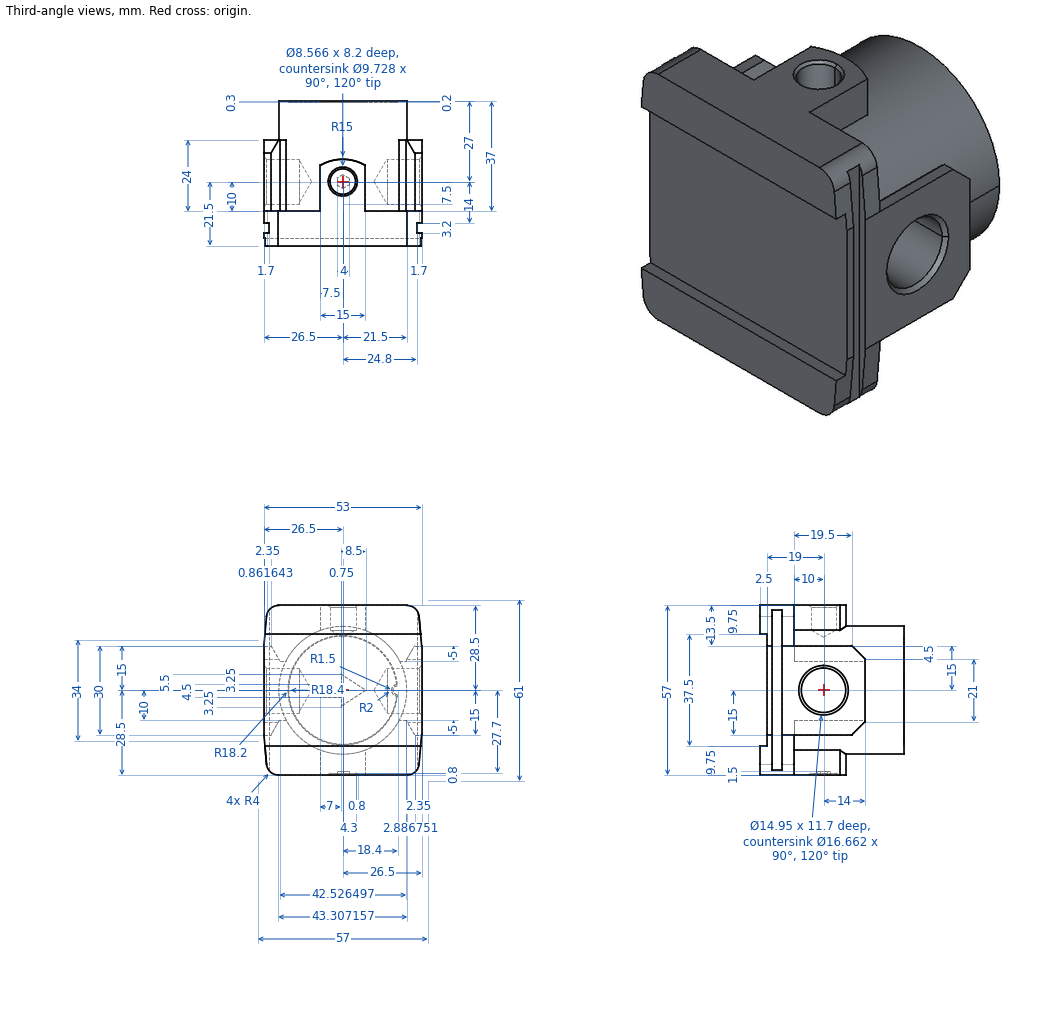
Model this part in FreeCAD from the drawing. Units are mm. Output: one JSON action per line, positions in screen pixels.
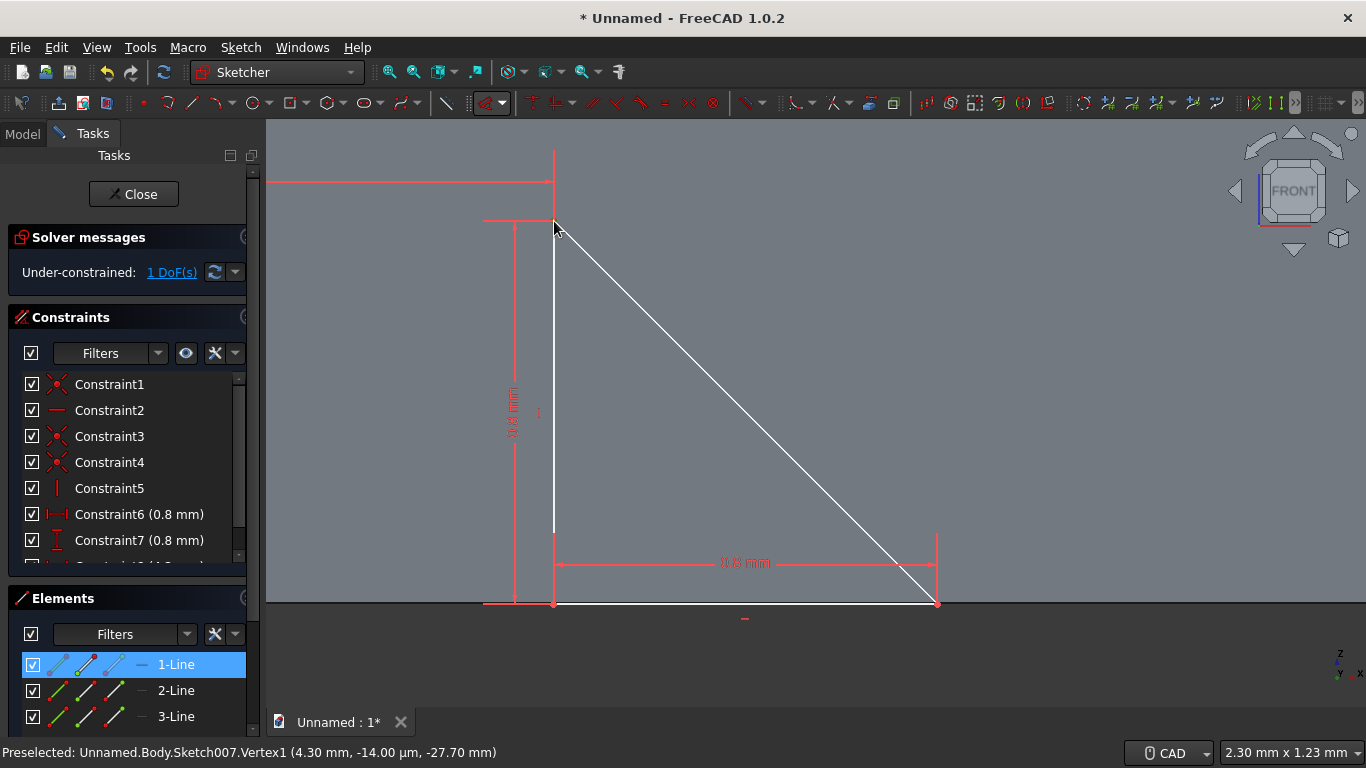
{"action": "left_click", "coordinate": [504, 104]}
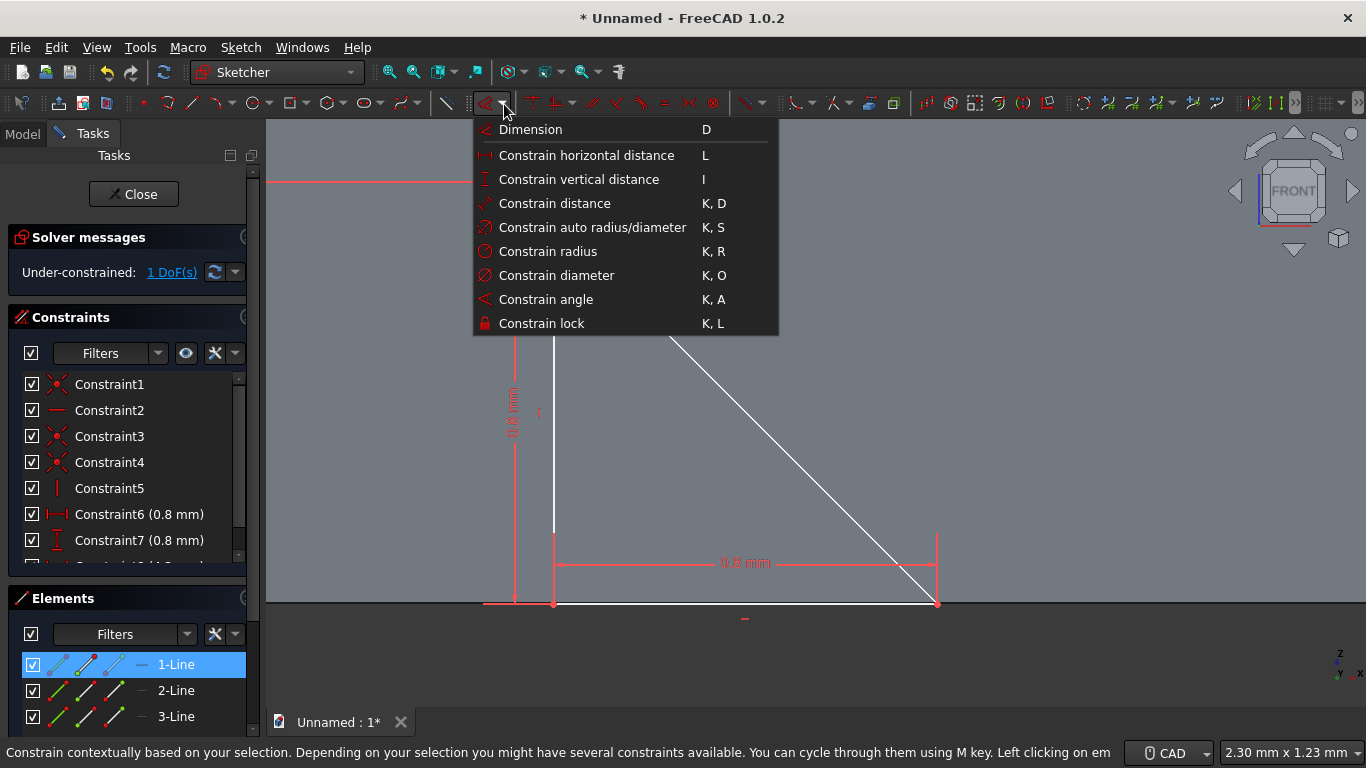
{"action": "left_click", "coordinate": [626, 179]}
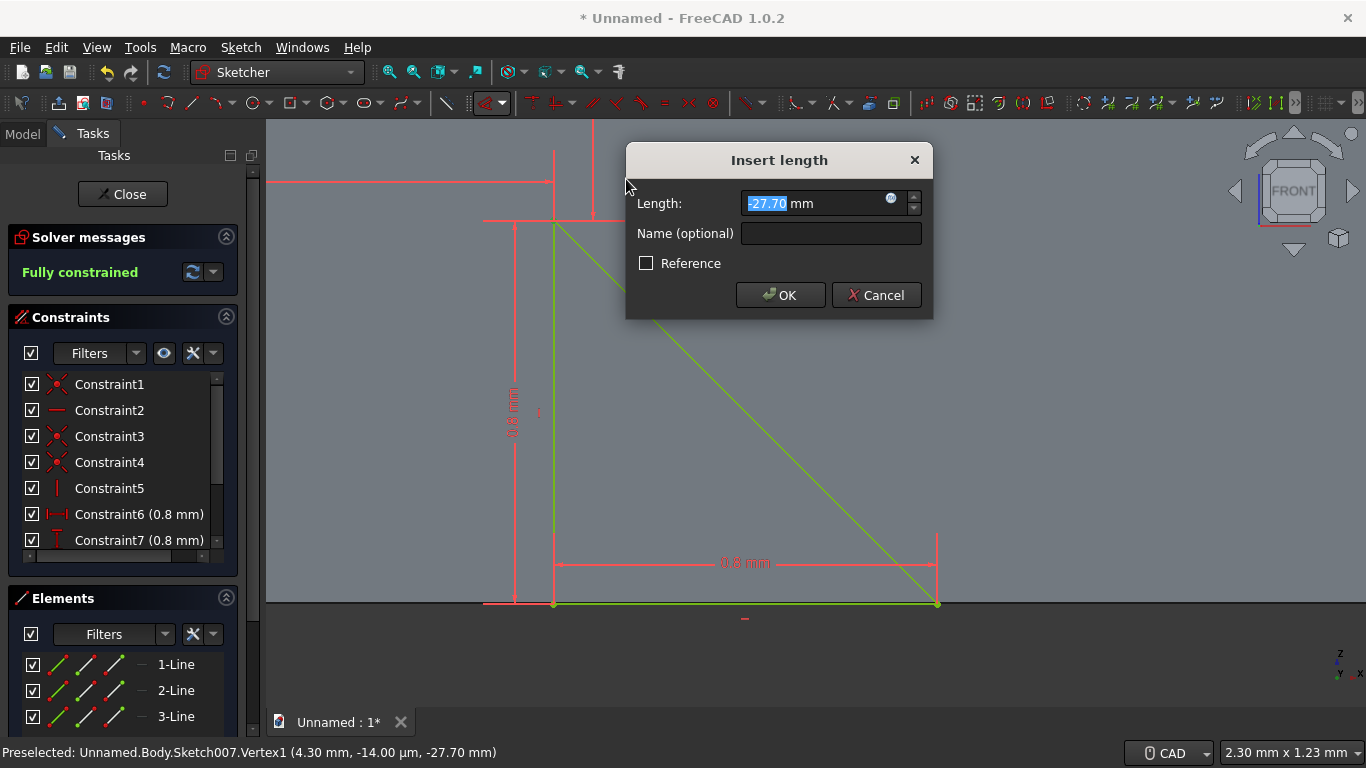
{"action": "type", "text": "-27.7"}
{"action": "key", "text": "Return"}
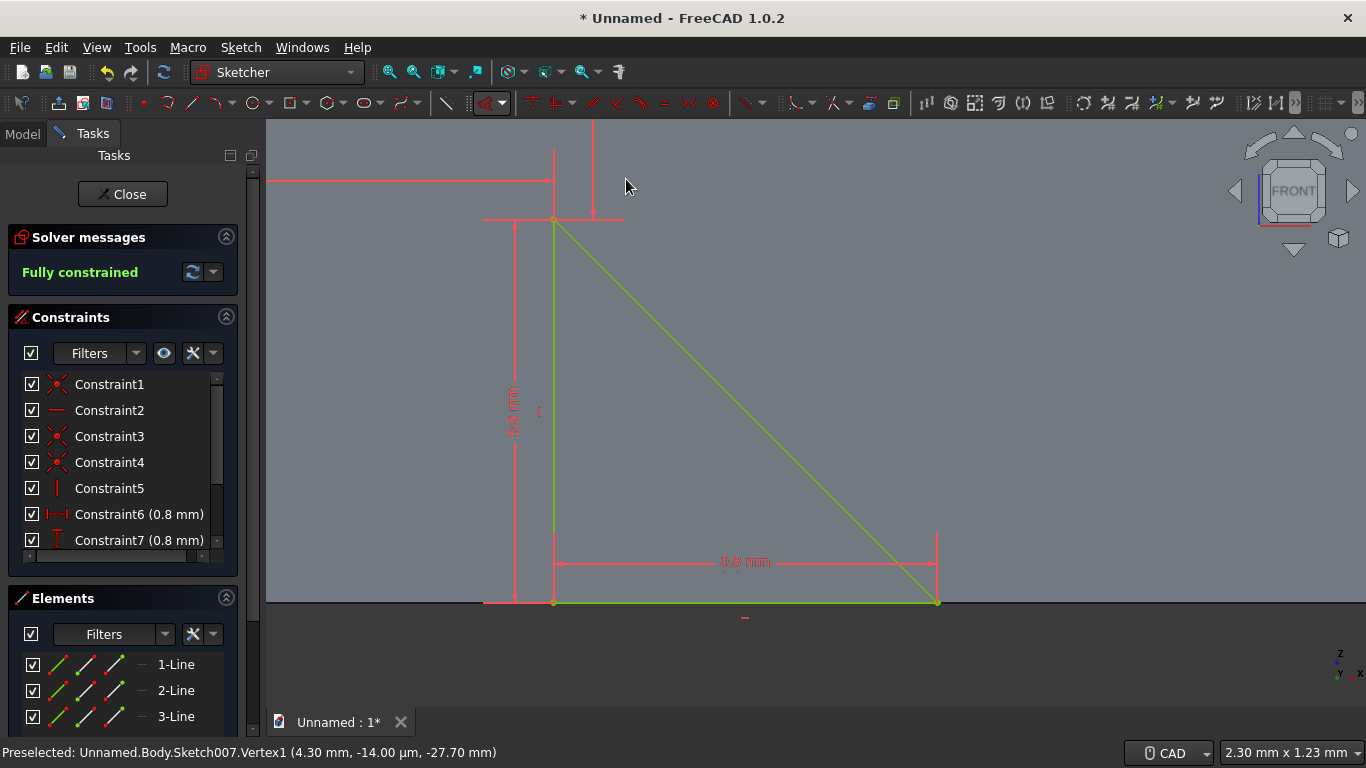
{"action": "left_click", "coordinate": [123, 194]}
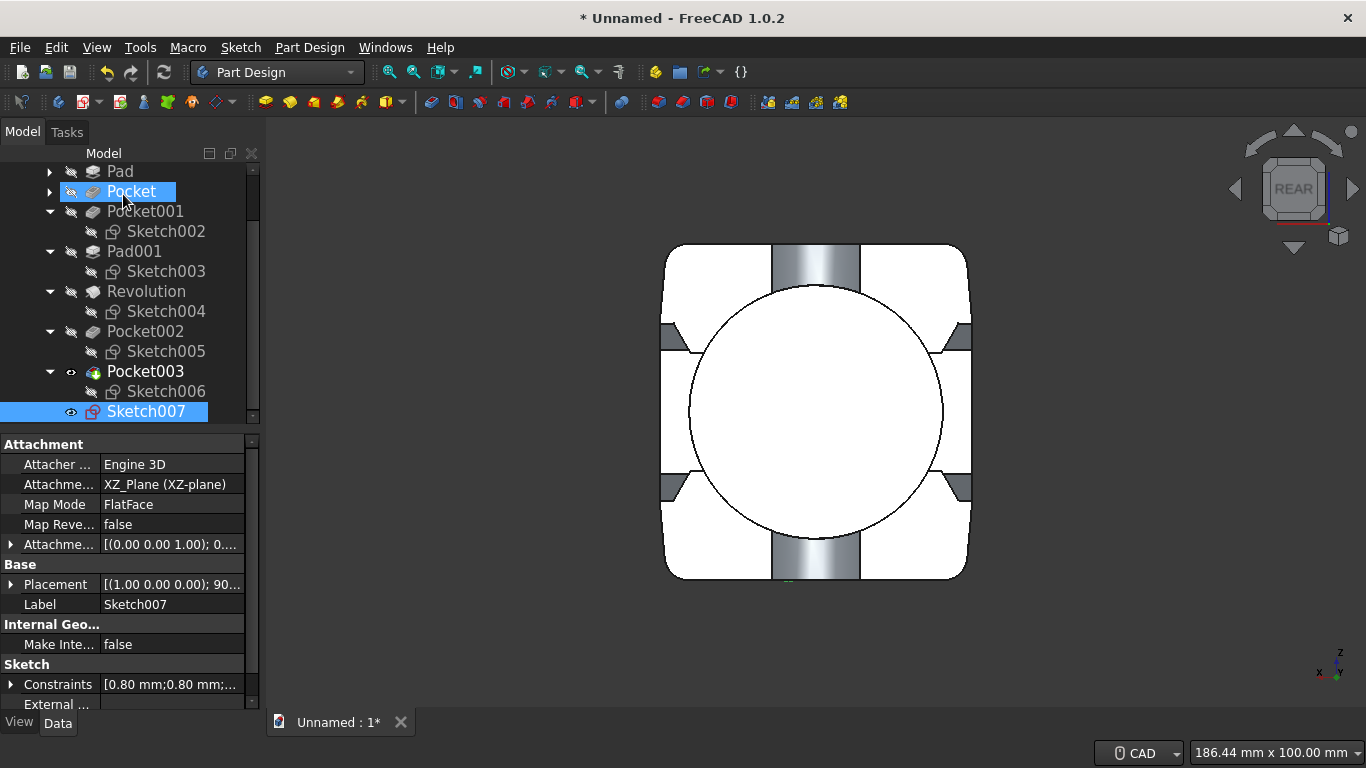
{"action": "left_click", "coordinate": [480, 102]}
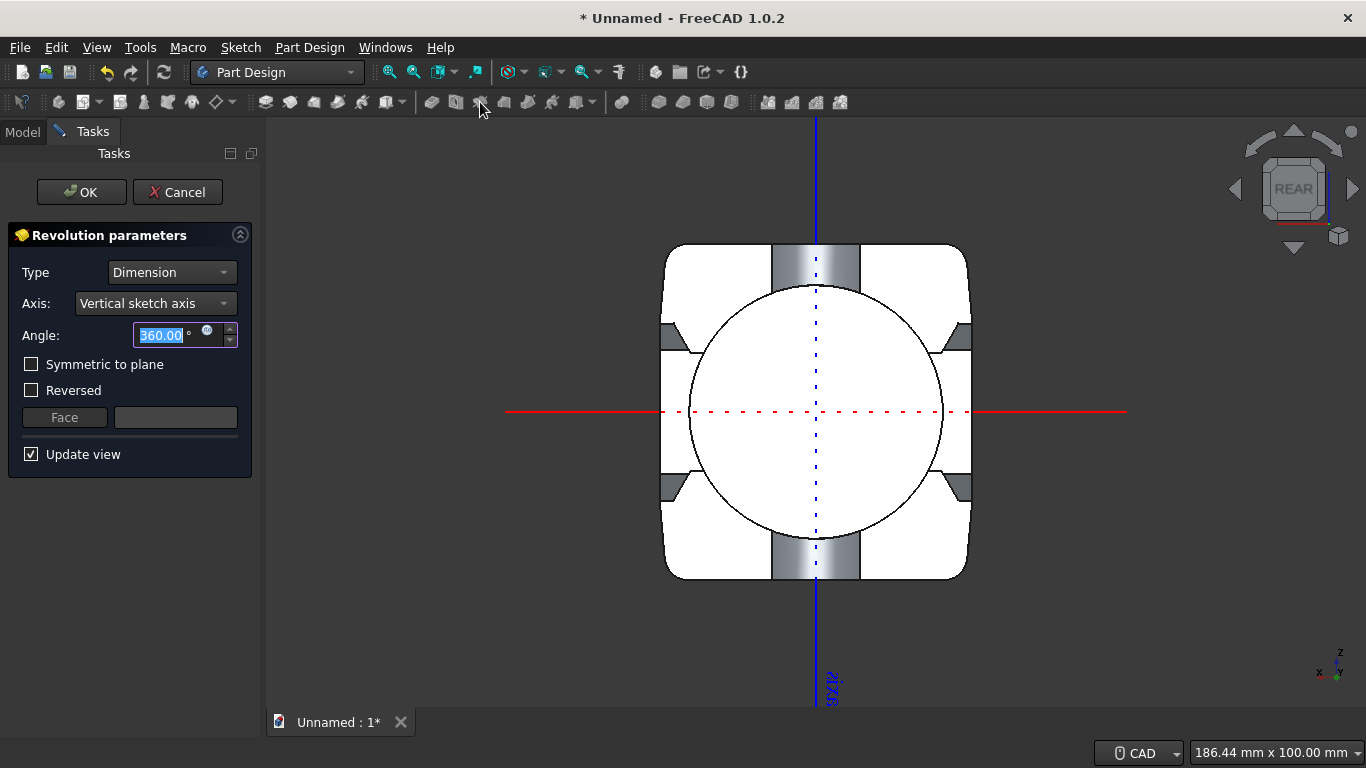
{"action": "left_click", "coordinate": [82, 192]}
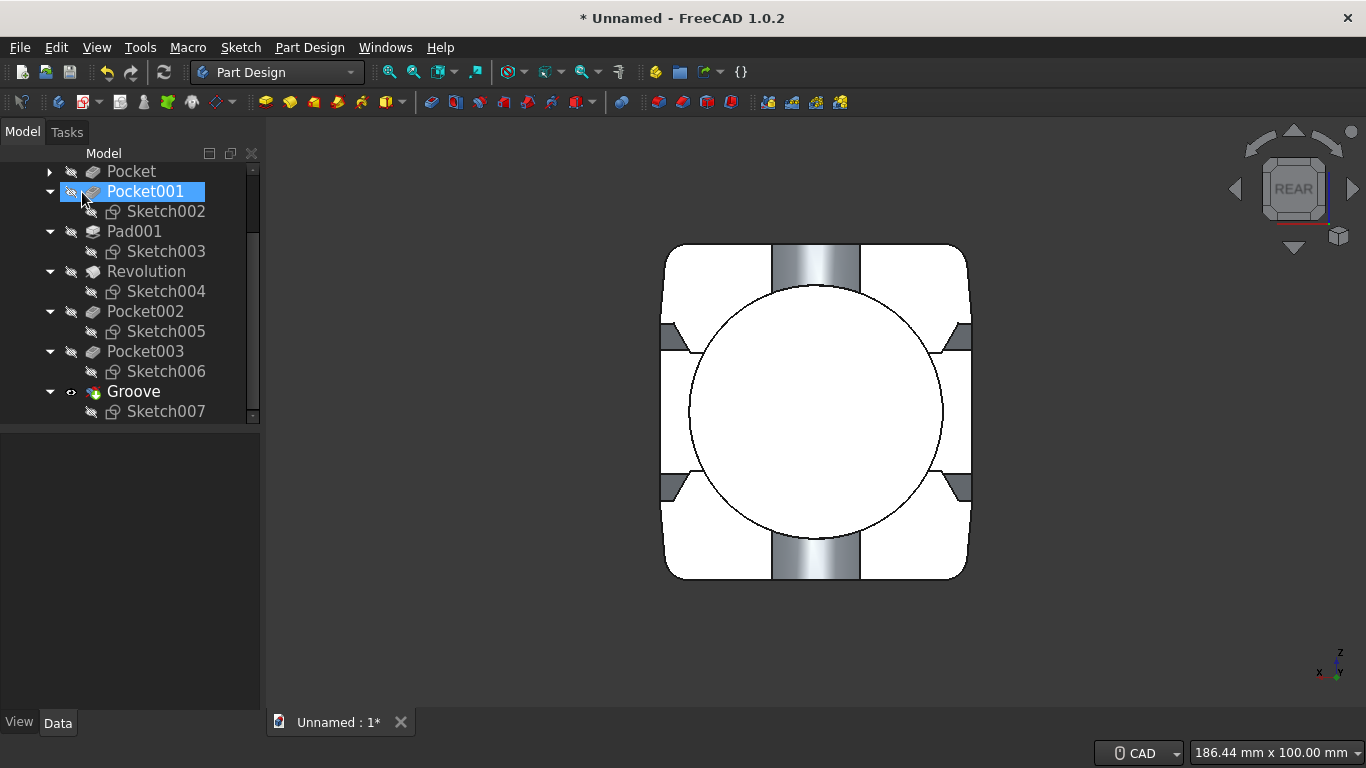
{"action": "key", "text": "0"}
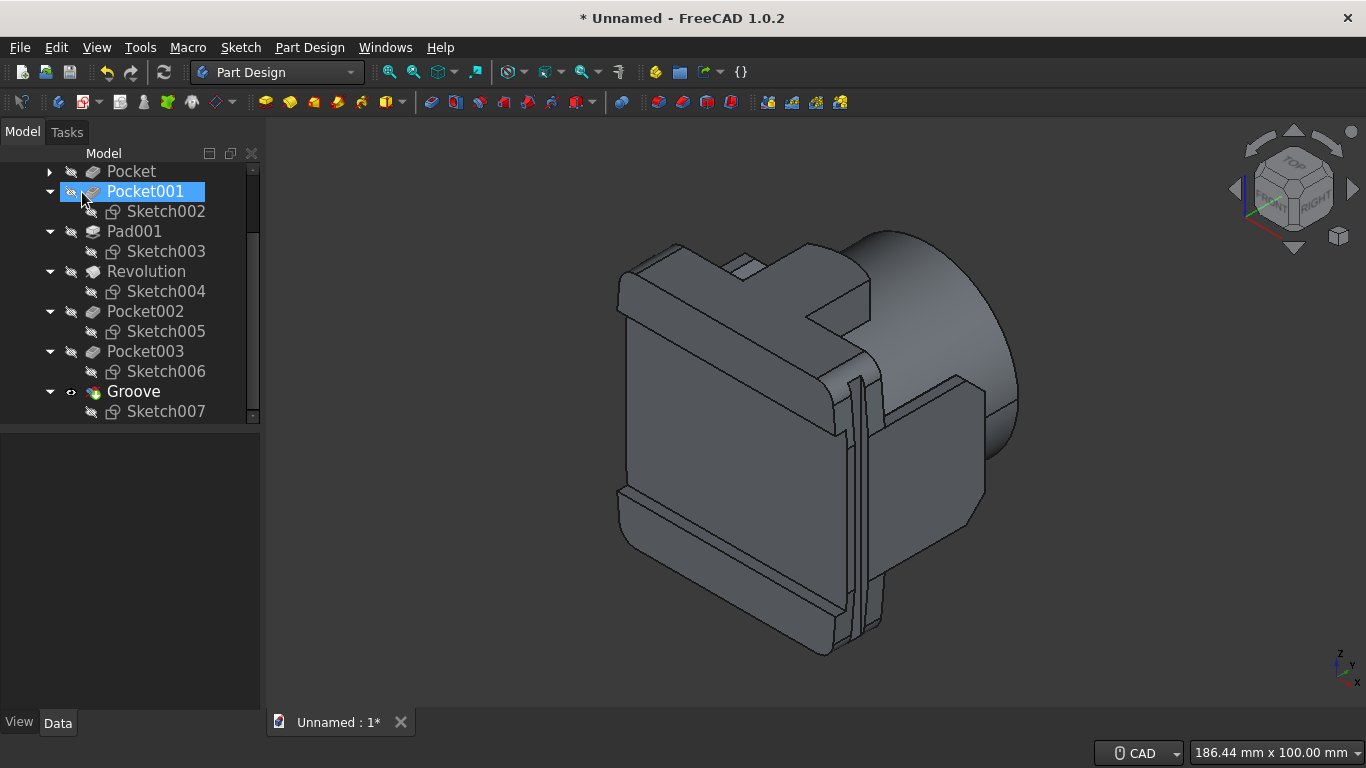
{"action": "left_click", "coordinate": [770, 301]}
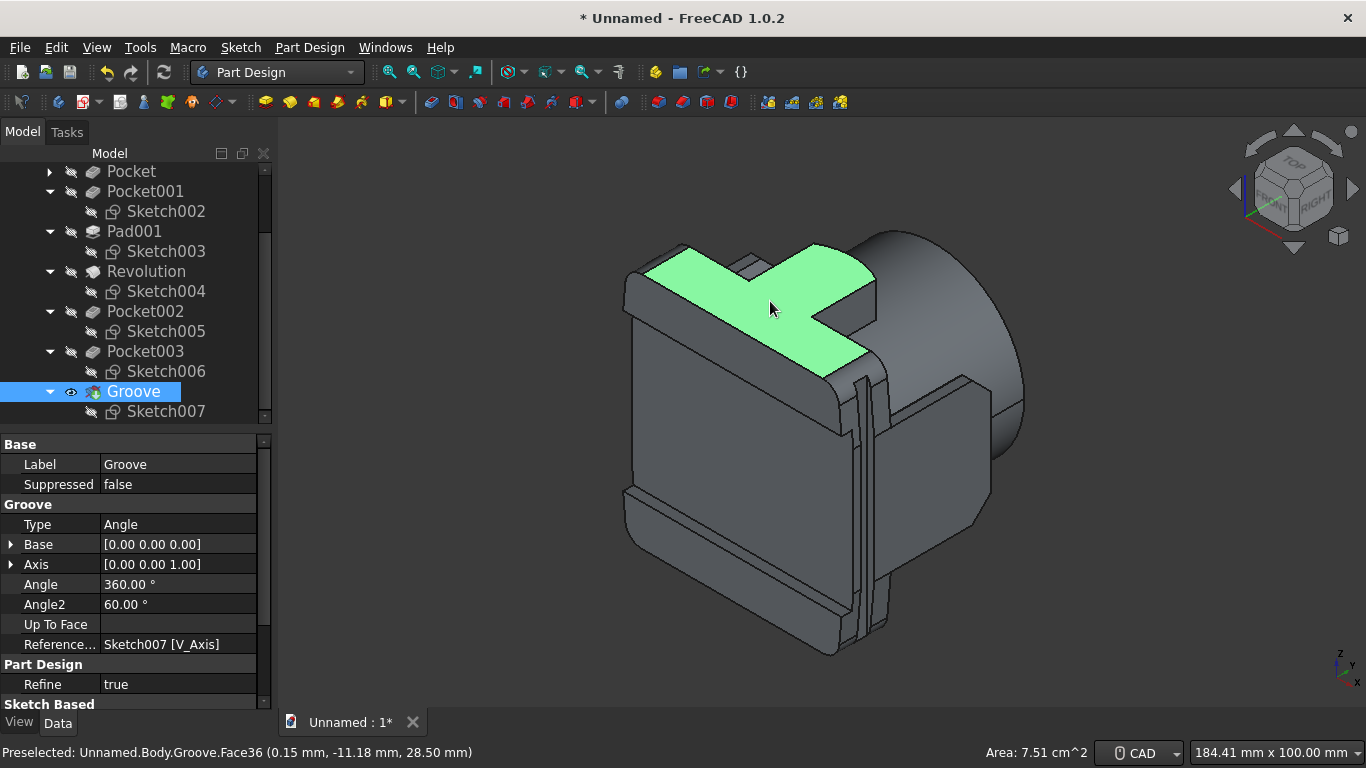
{"action": "left_click", "coordinate": [84, 102]}